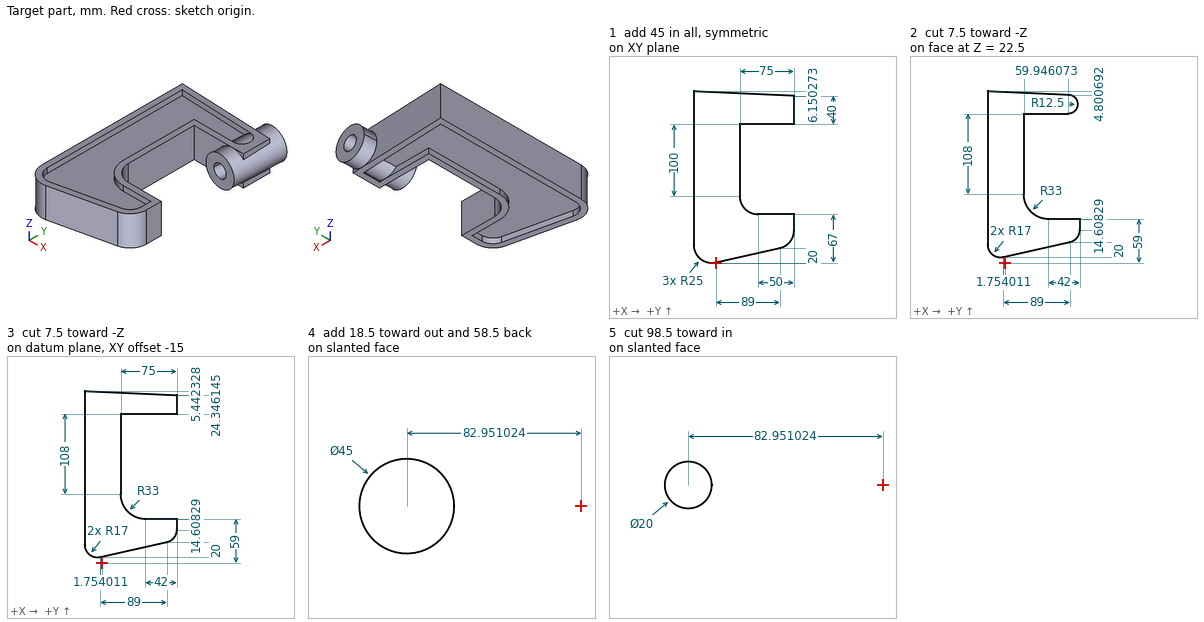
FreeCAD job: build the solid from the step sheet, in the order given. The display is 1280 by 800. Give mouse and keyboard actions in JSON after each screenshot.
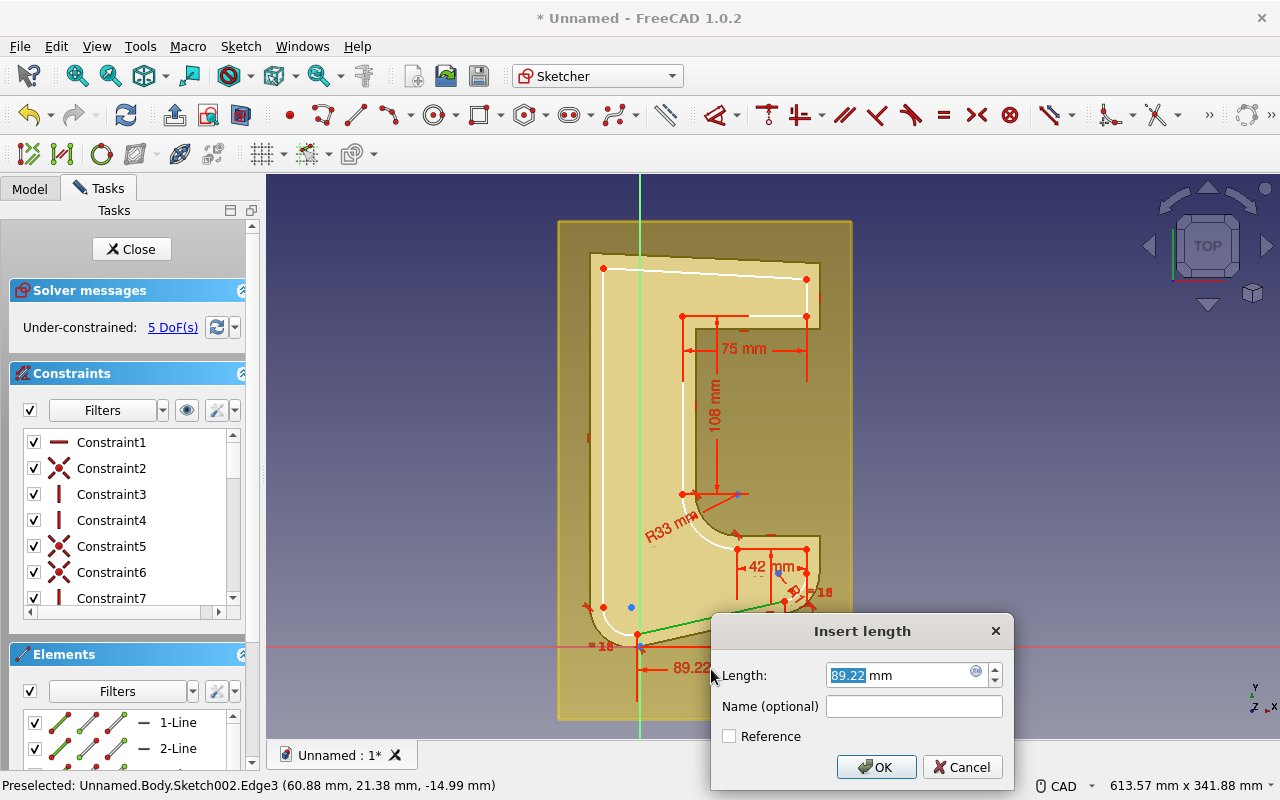
{"action": "type", "text": "89"}
{"action": "key", "text": "Return"}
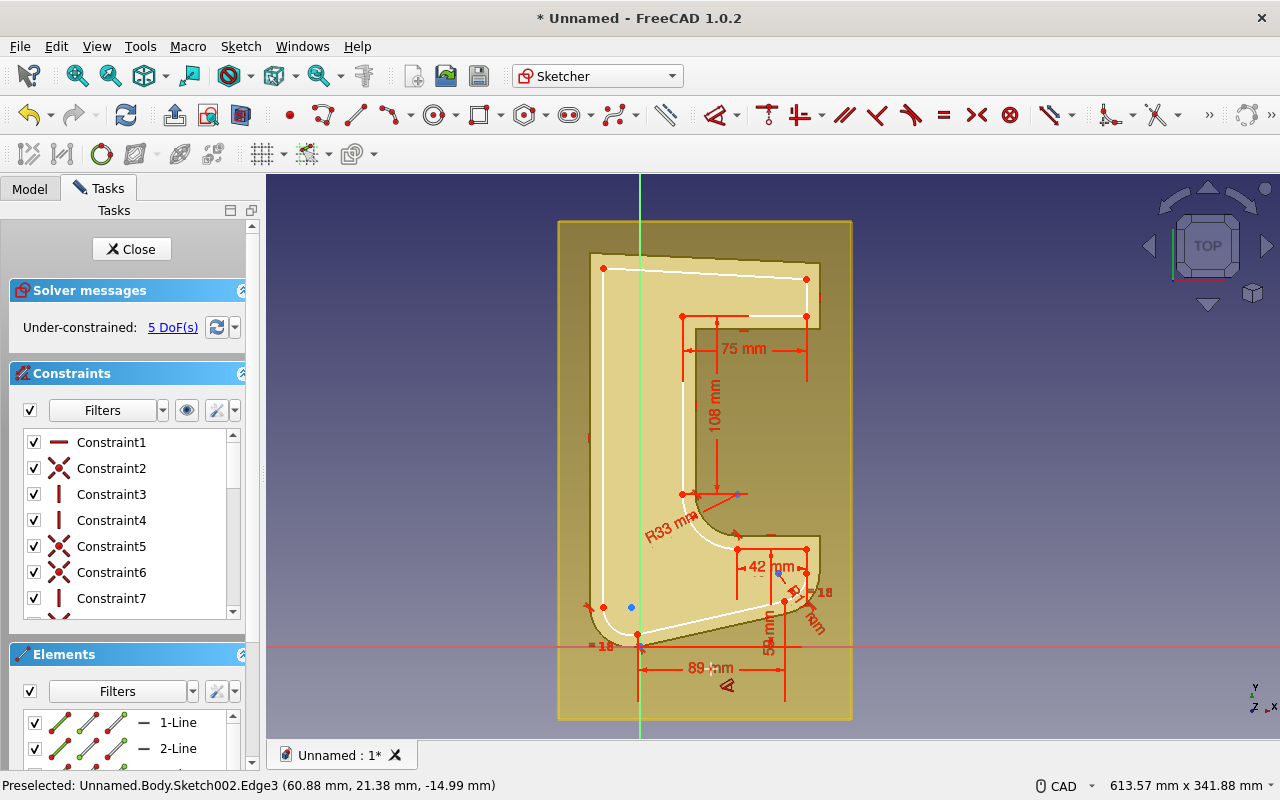
{"action": "left_click", "coordinate": [741, 611]}
{"action": "left_click", "coordinate": [580, 618]}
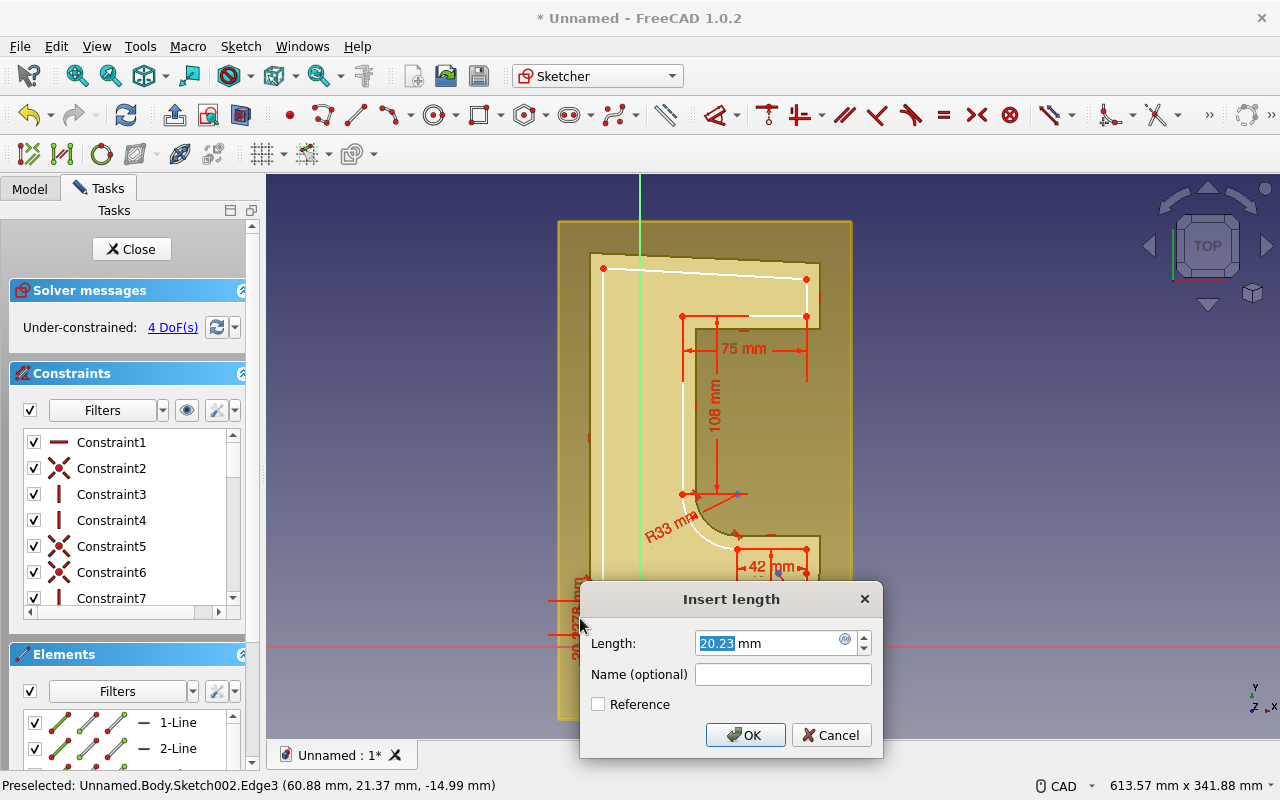
{"action": "type", "text": "20"}
{"action": "key", "text": "Return"}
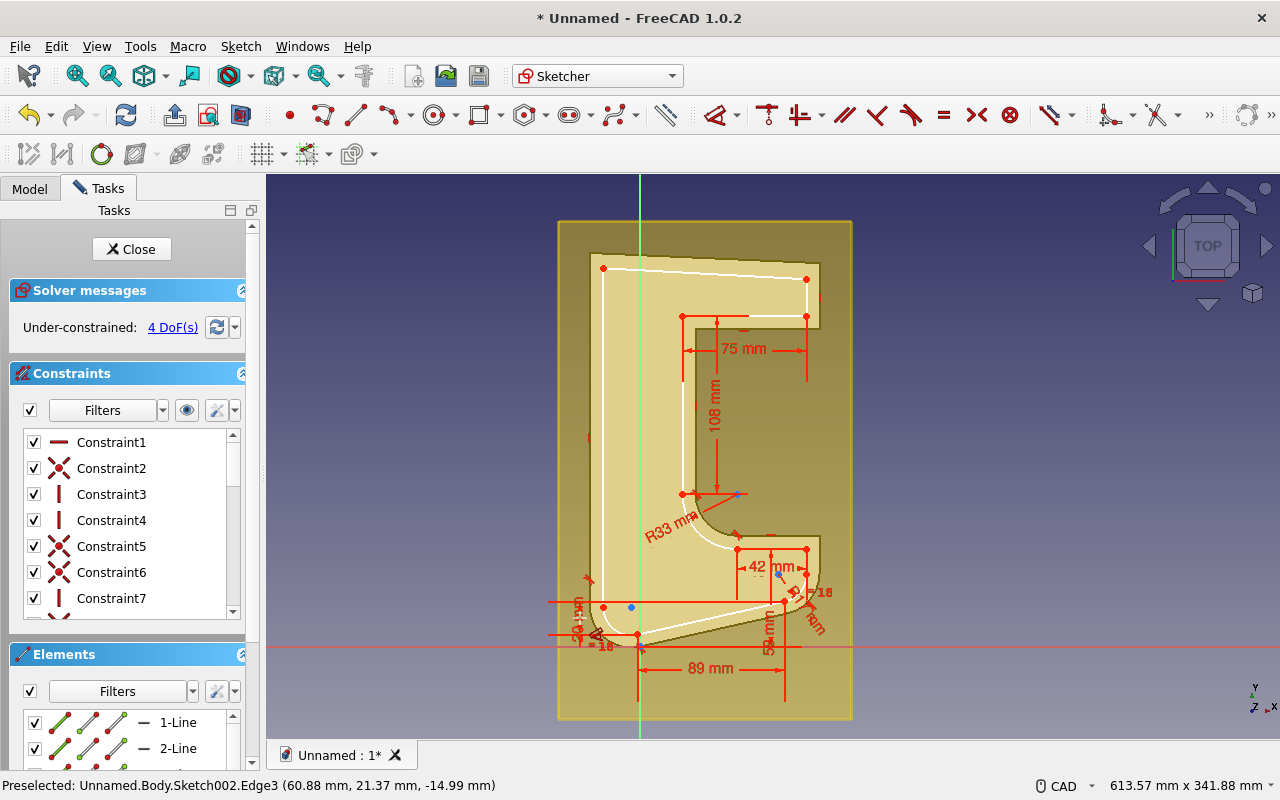
{"action": "scroll", "coordinate": [807, 559], "scroll_direction": "up", "scroll_amount": 3}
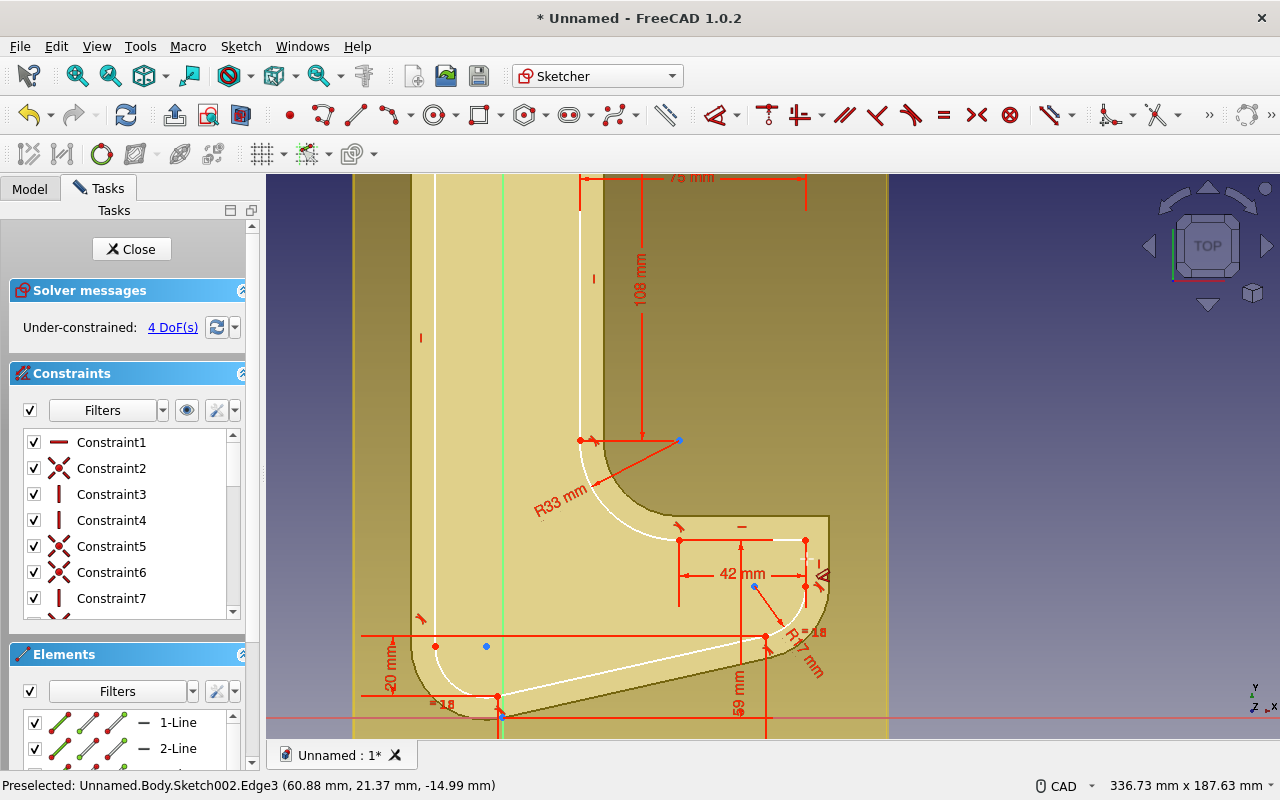
{"action": "left_click", "coordinate": [806, 559]}
{"action": "left_click", "coordinate": [840, 563]}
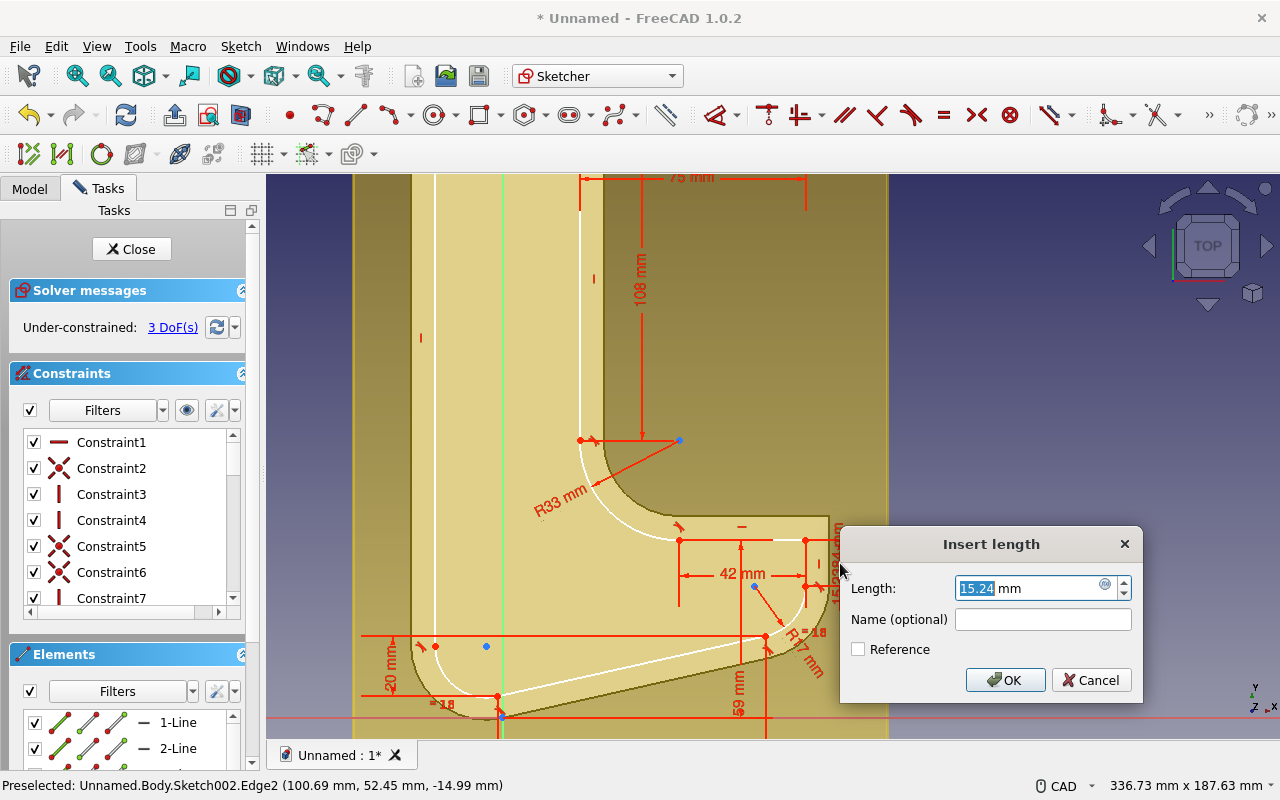
{"action": "type", "text": "14.60829"}
{"action": "key", "text": "Return"}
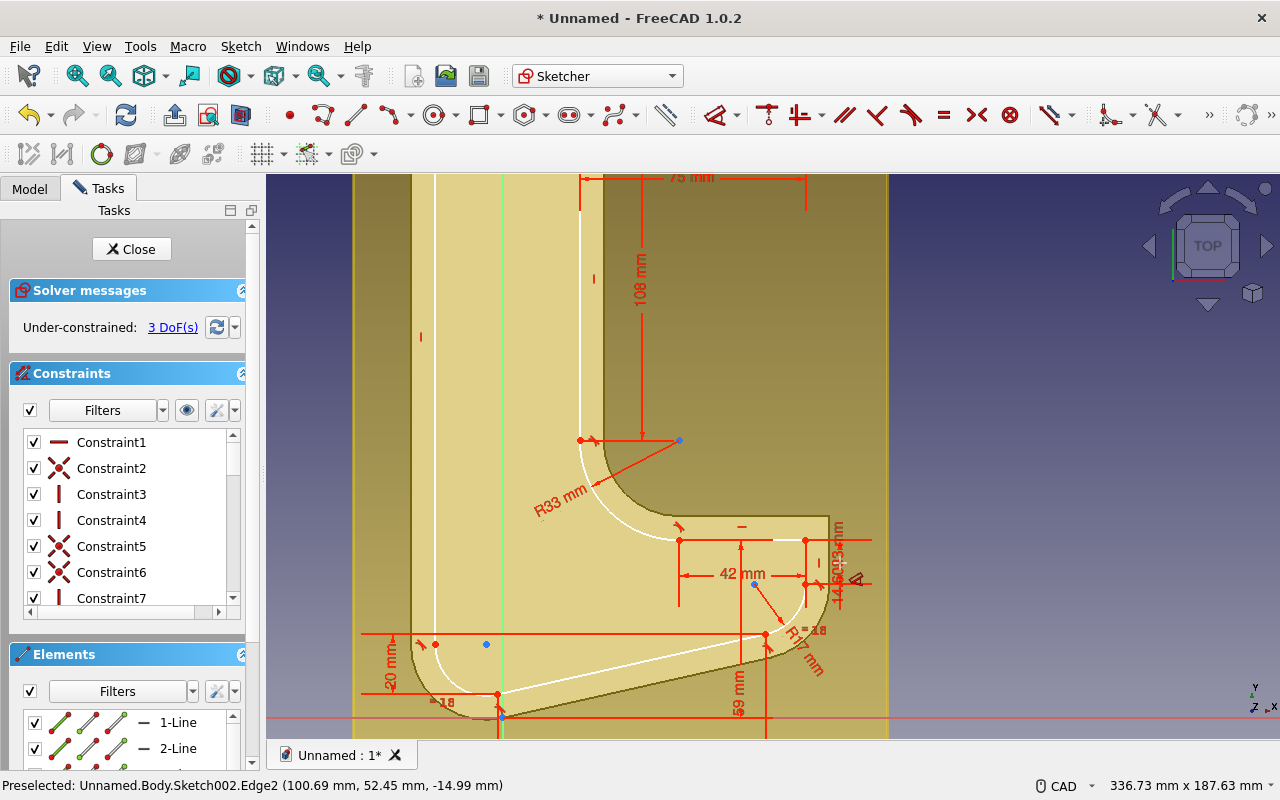
{"action": "scroll", "coordinate": [807, 559], "scroll_direction": "down", "scroll_amount": 3}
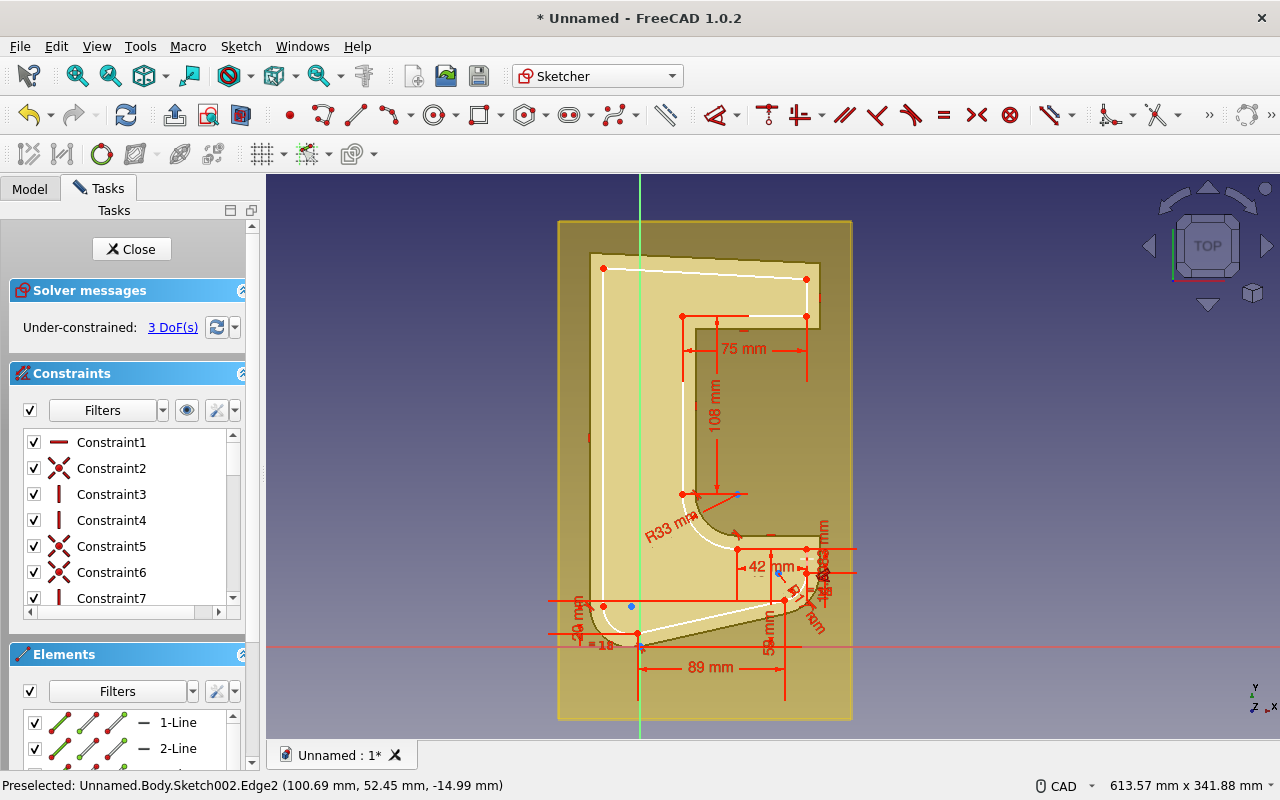
{"action": "scroll", "coordinate": [807, 290], "scroll_direction": "up", "scroll_amount": 2}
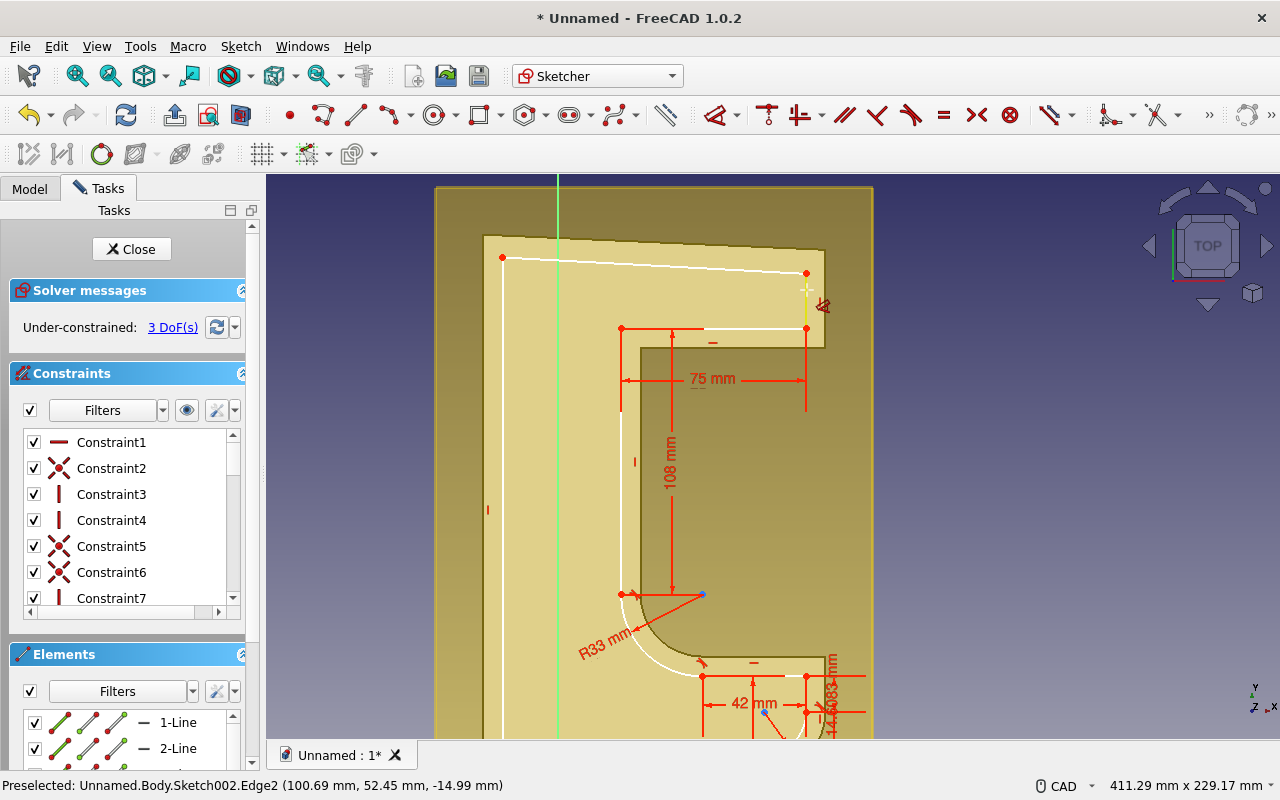
{"action": "left_click", "coordinate": [806, 290]}
{"action": "left_click", "coordinate": [840, 301]}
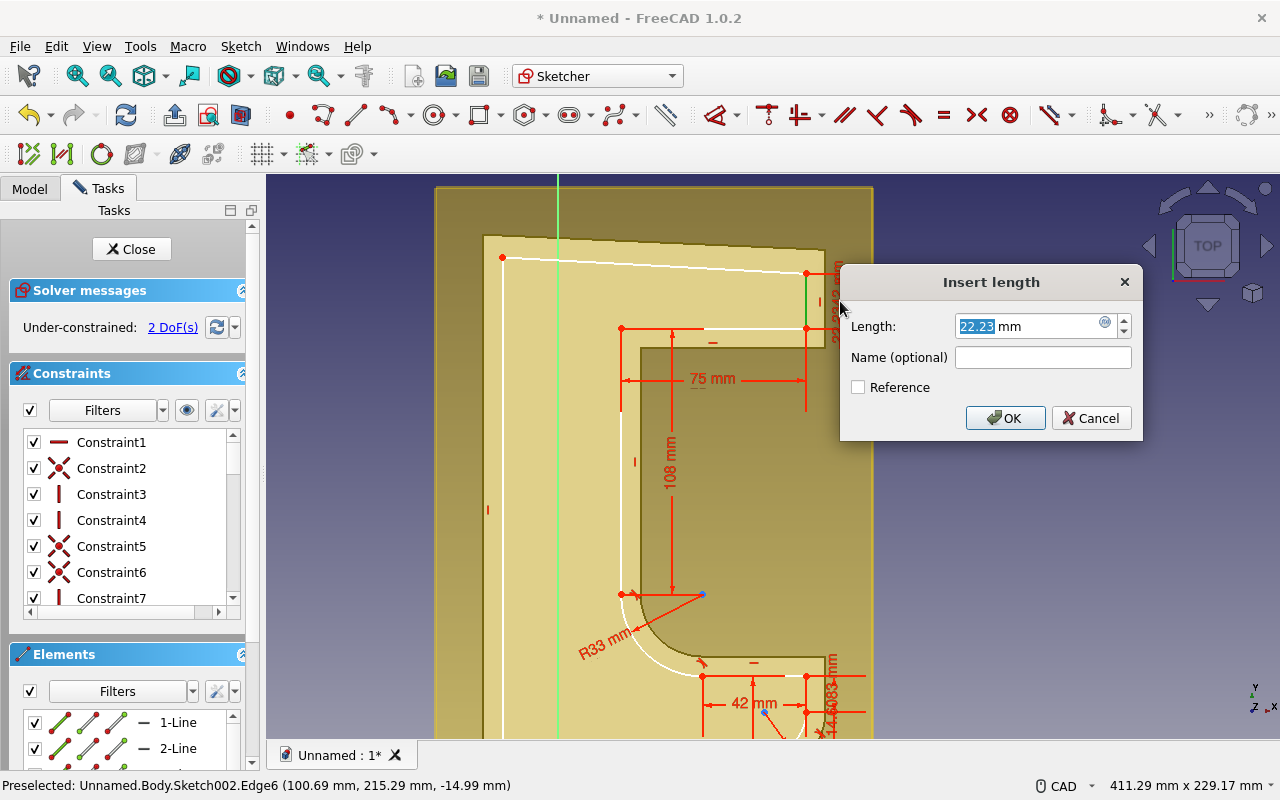
{"action": "type", "text": "24.346145"}
{"action": "key", "text": "Return"}